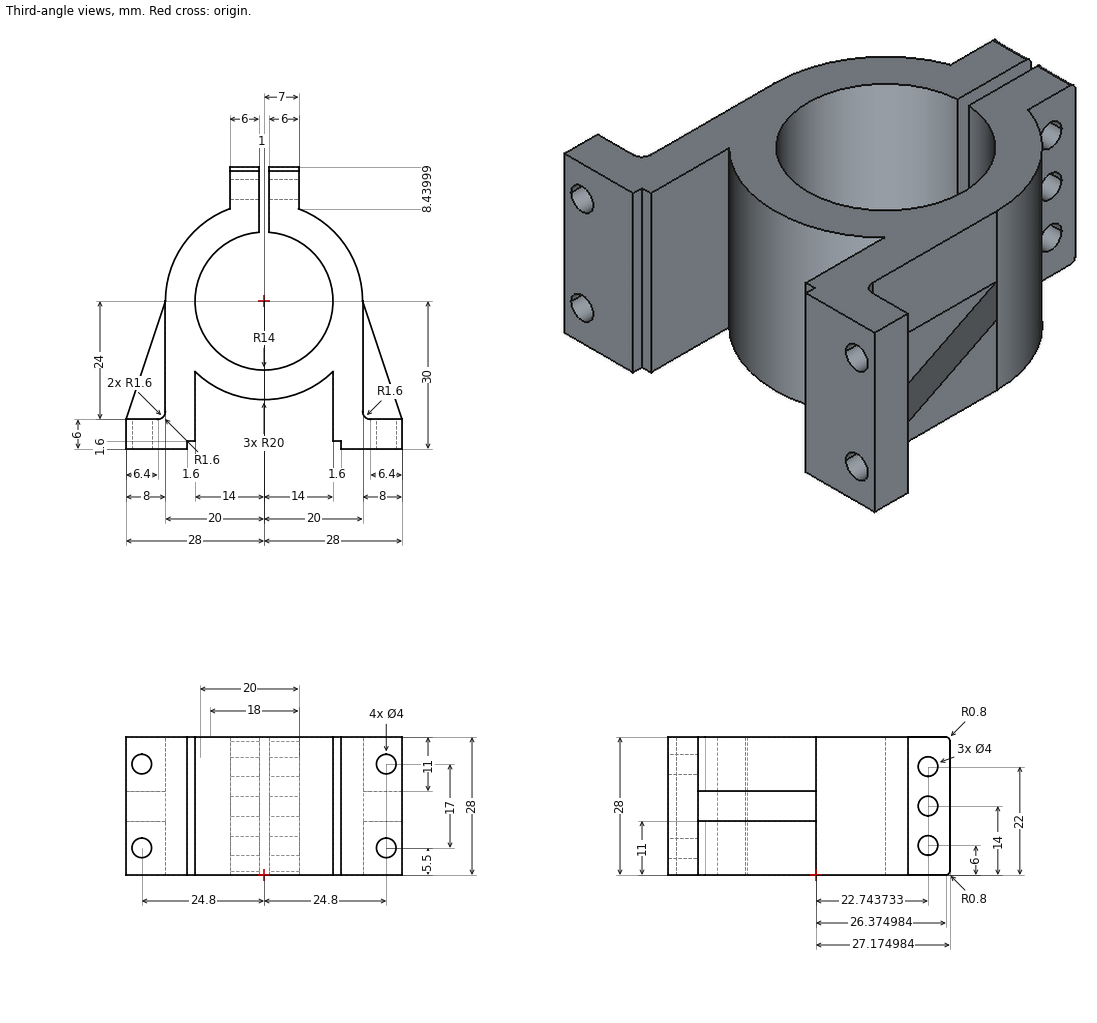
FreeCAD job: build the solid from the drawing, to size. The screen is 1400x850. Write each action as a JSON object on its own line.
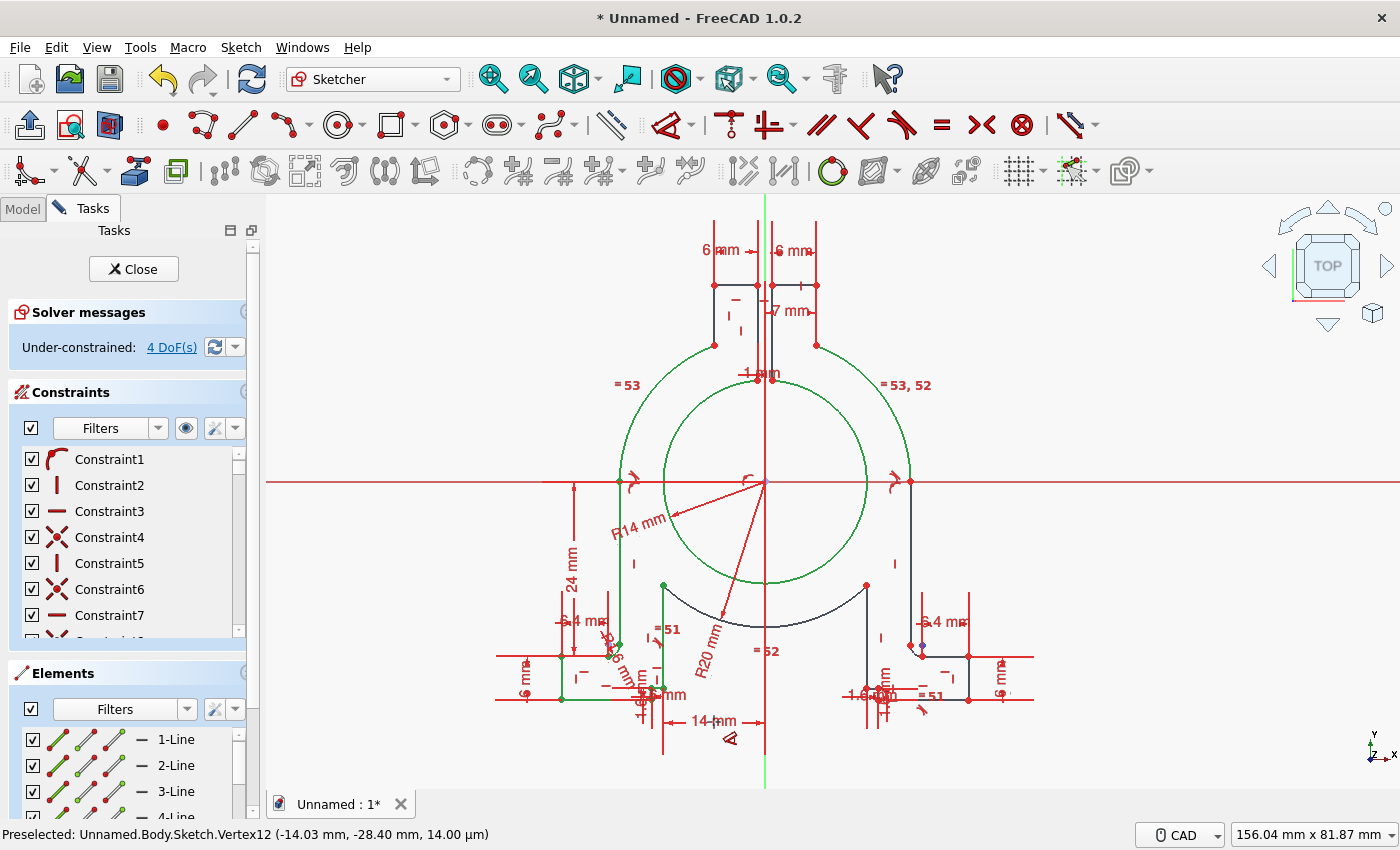
{"action": "left_click", "coordinate": [867, 586]}
{"action": "left_click", "coordinate": [852, 620]}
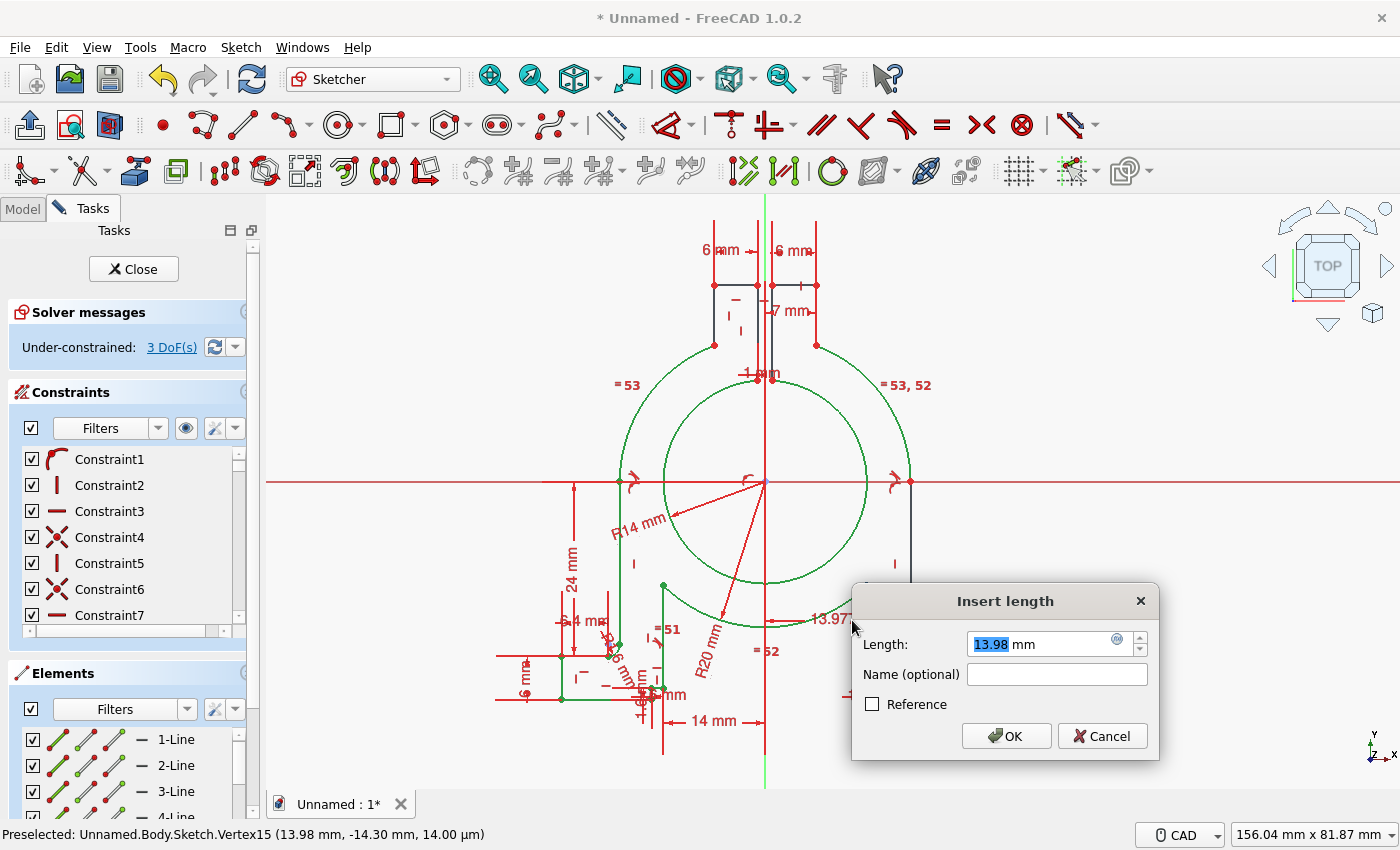
{"action": "type", "text": "14"}
{"action": "key", "text": "Return"}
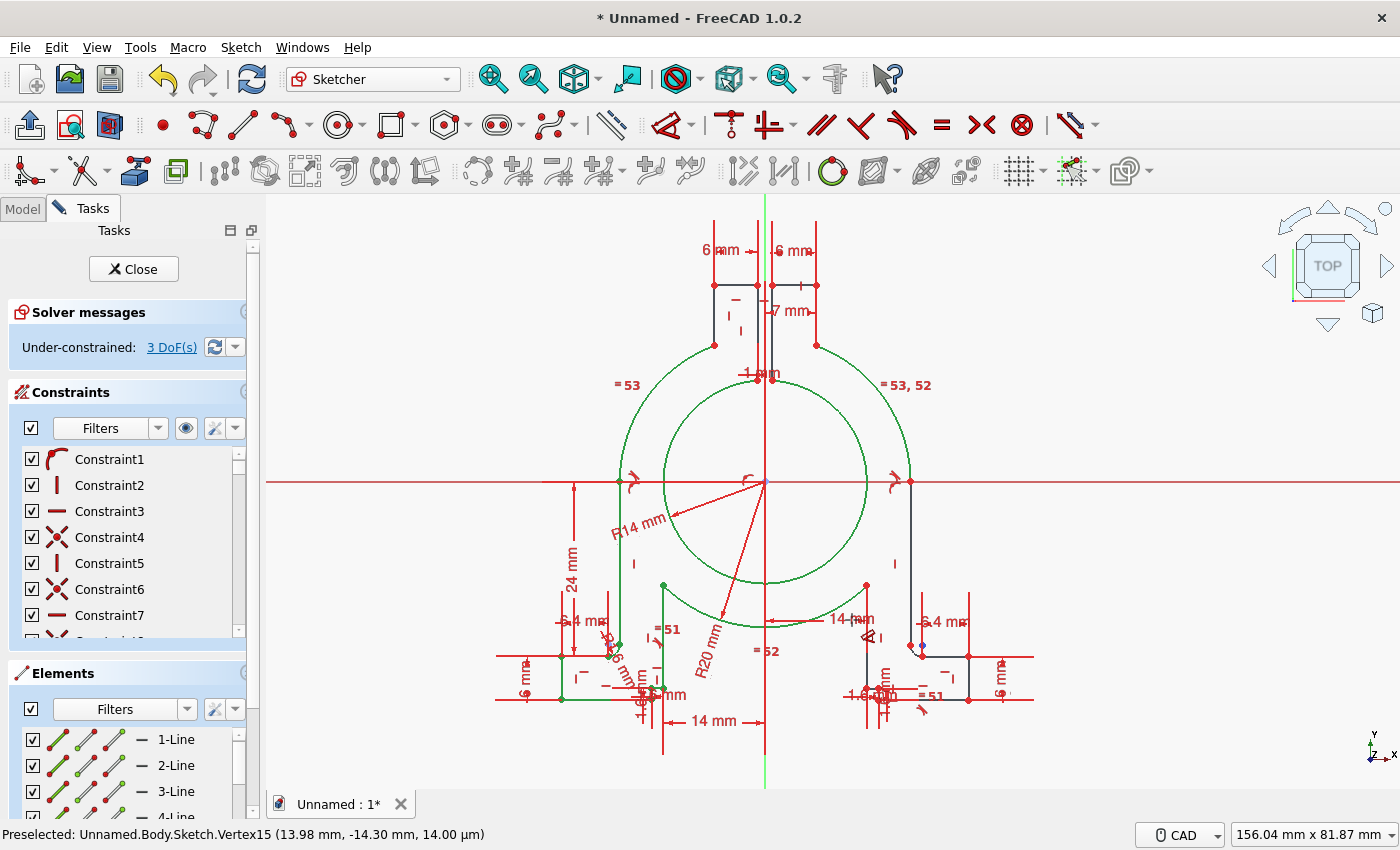
{"action": "left_click", "coordinate": [879, 700]}
{"action": "left_click", "coordinate": [731, 541]}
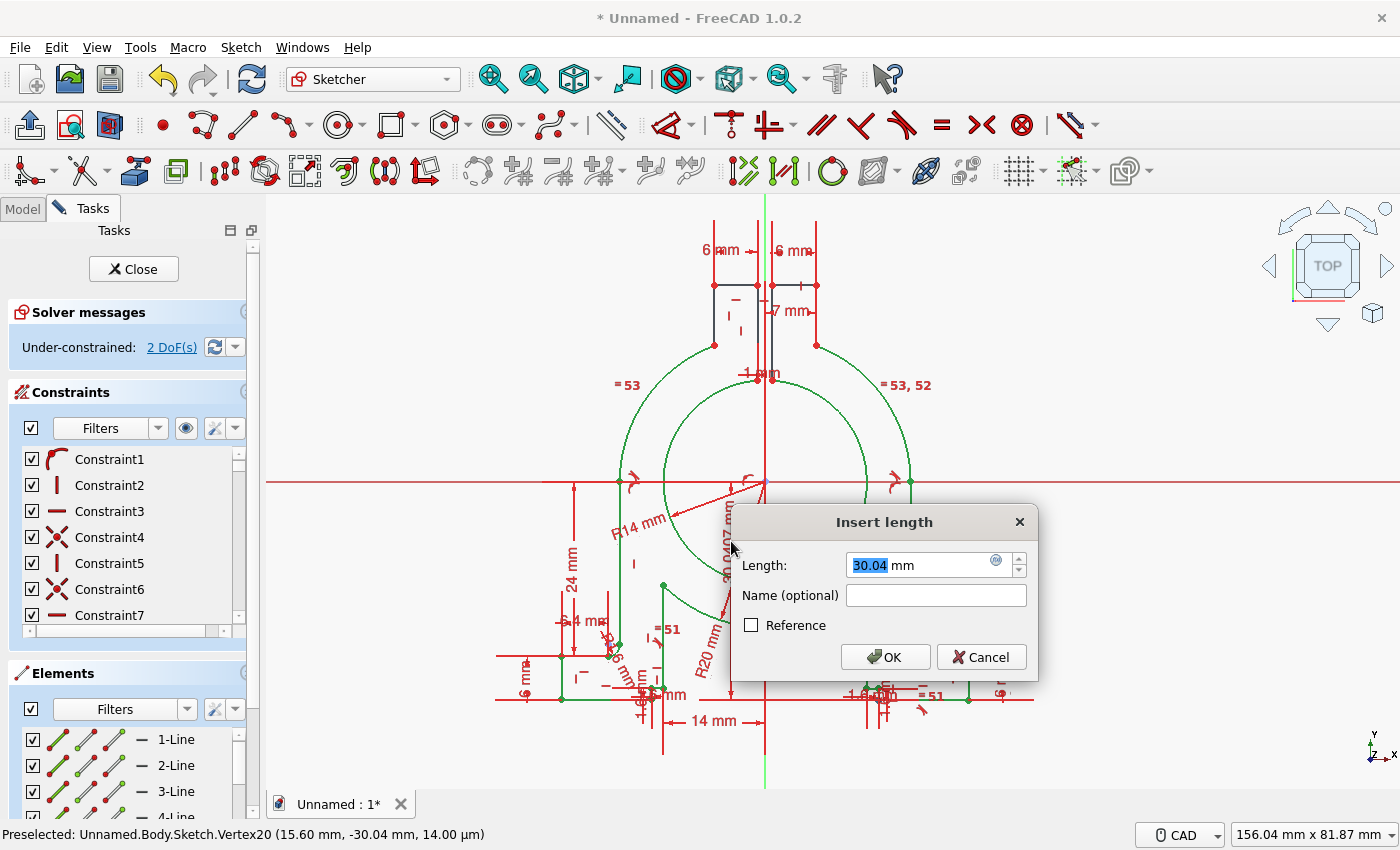
{"action": "type", "text": "30"}
{"action": "key", "text": "Return"}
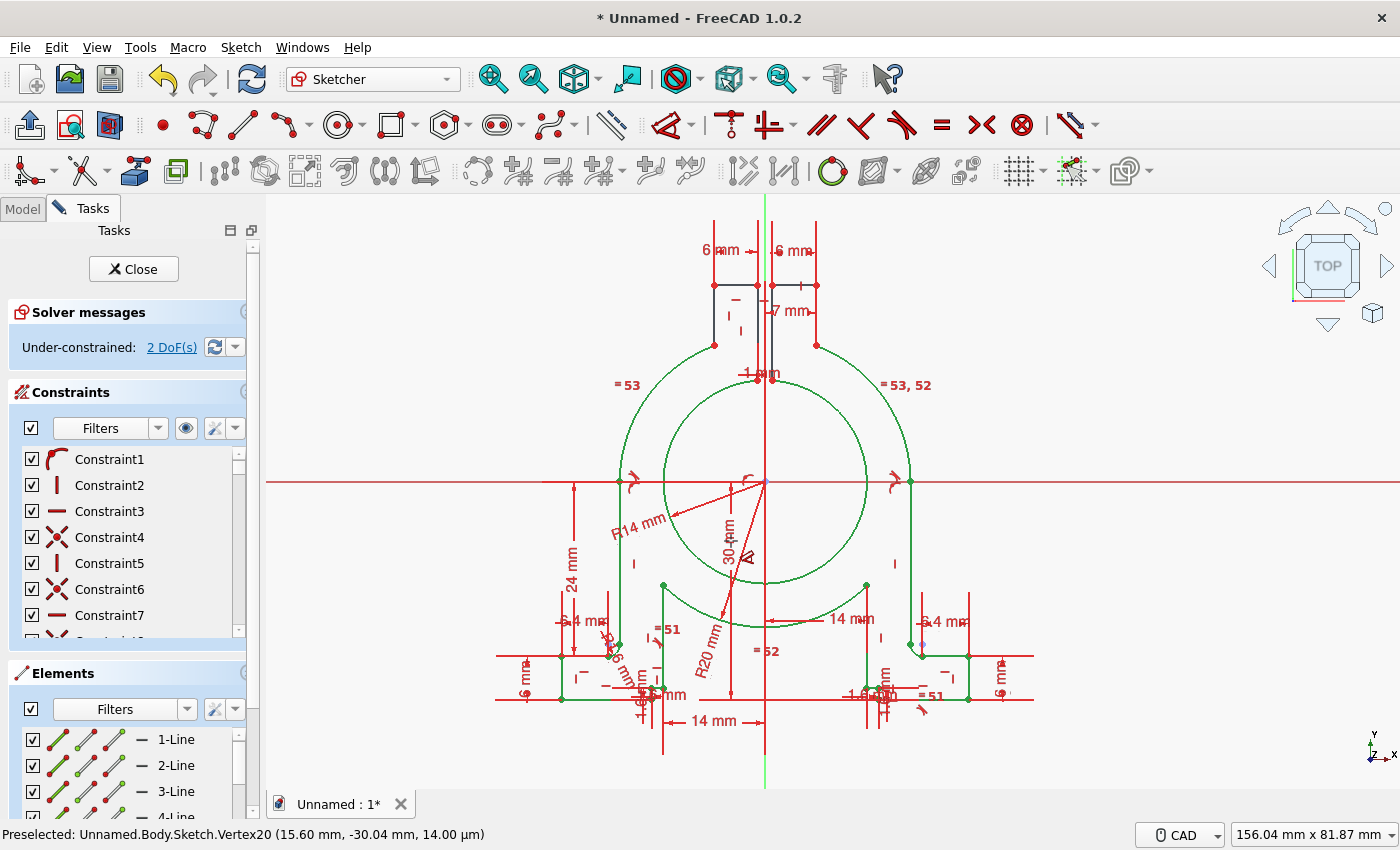
{"action": "left_click", "coordinate": [816, 328]}
{"action": "left_click", "coordinate": [850, 337]}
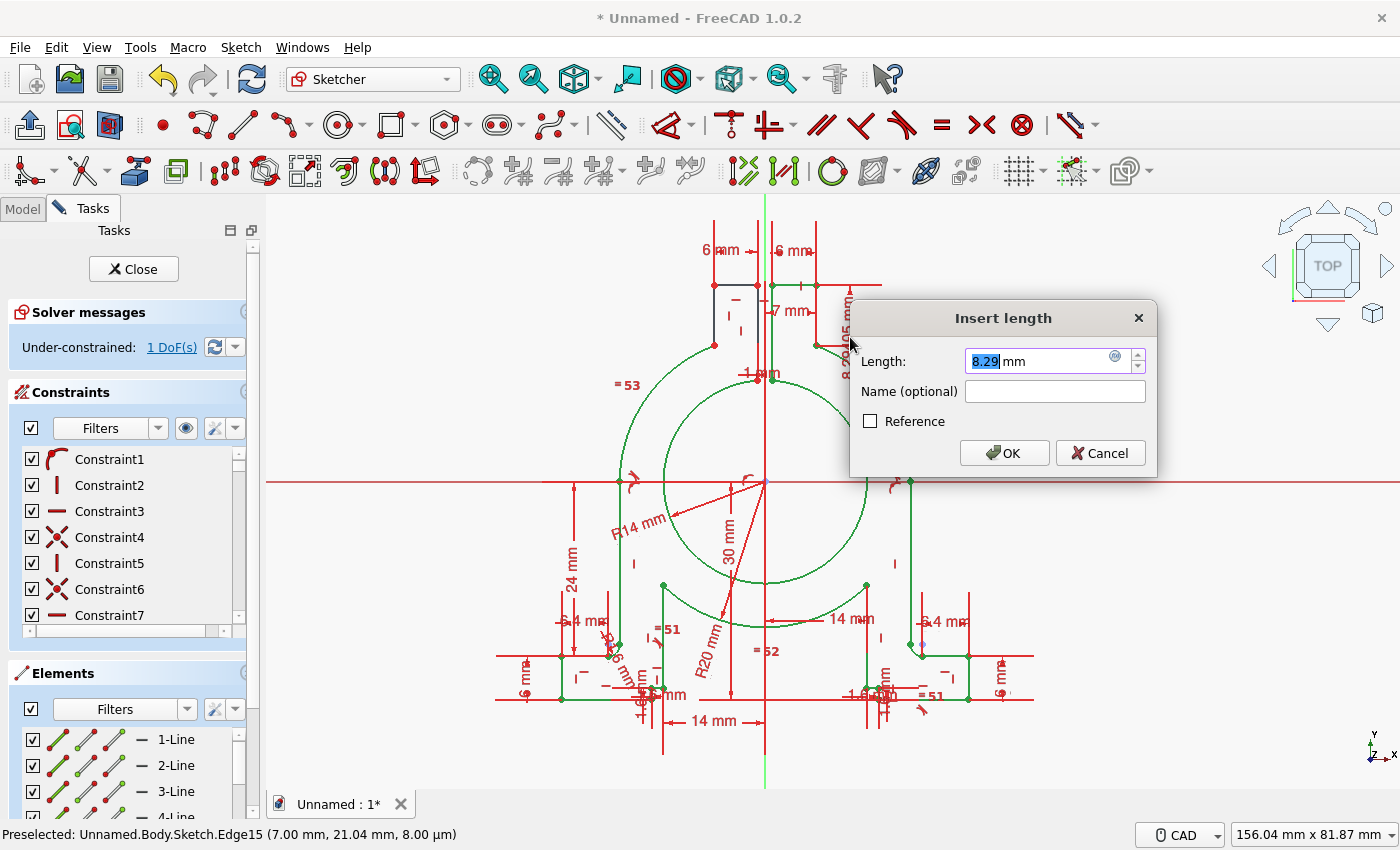
{"action": "type", "text": "8.43999"}
{"action": "key", "text": "Return"}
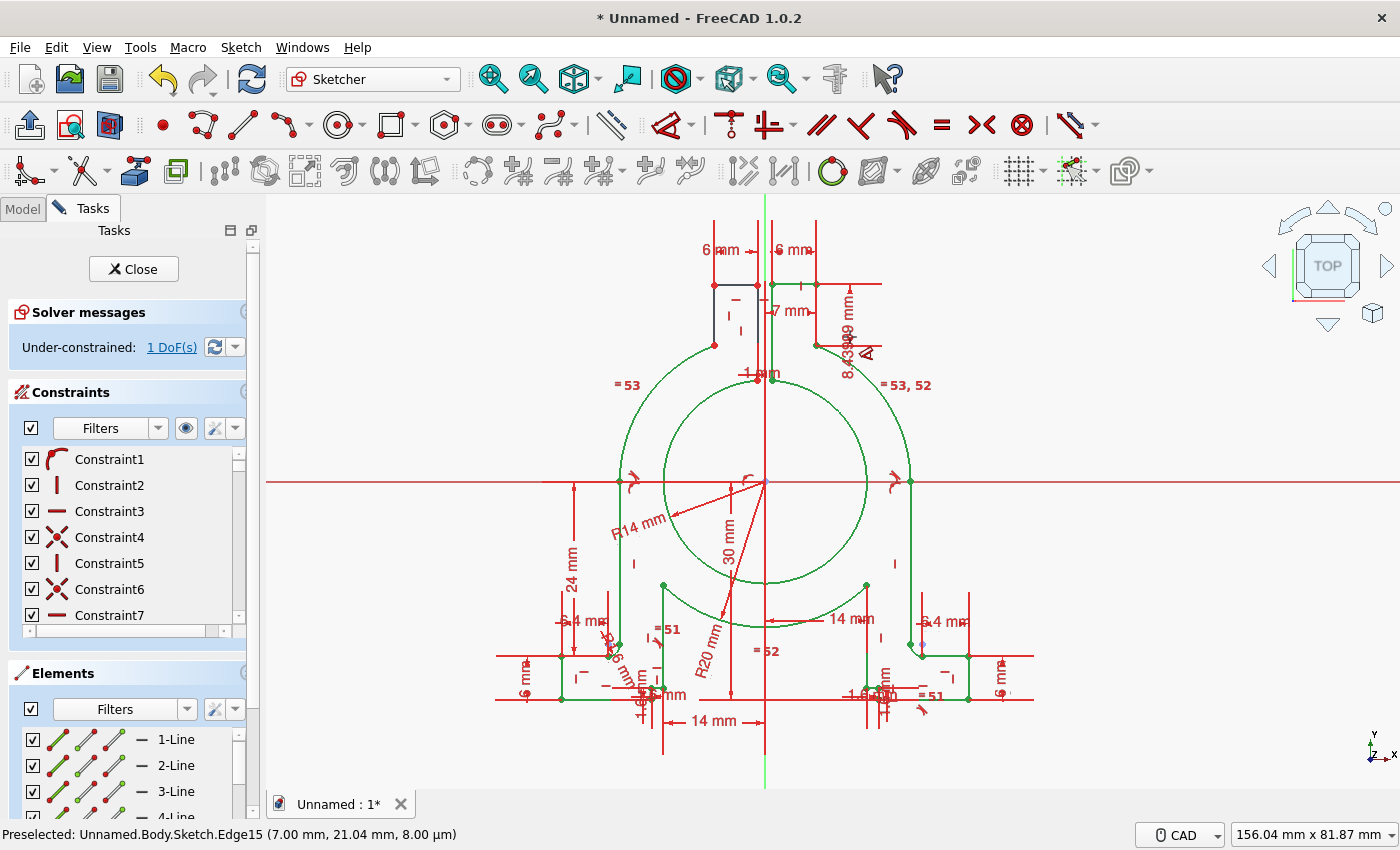
{"action": "left_click", "coordinate": [714, 303]}
{"action": "left_click", "coordinate": [680, 315]}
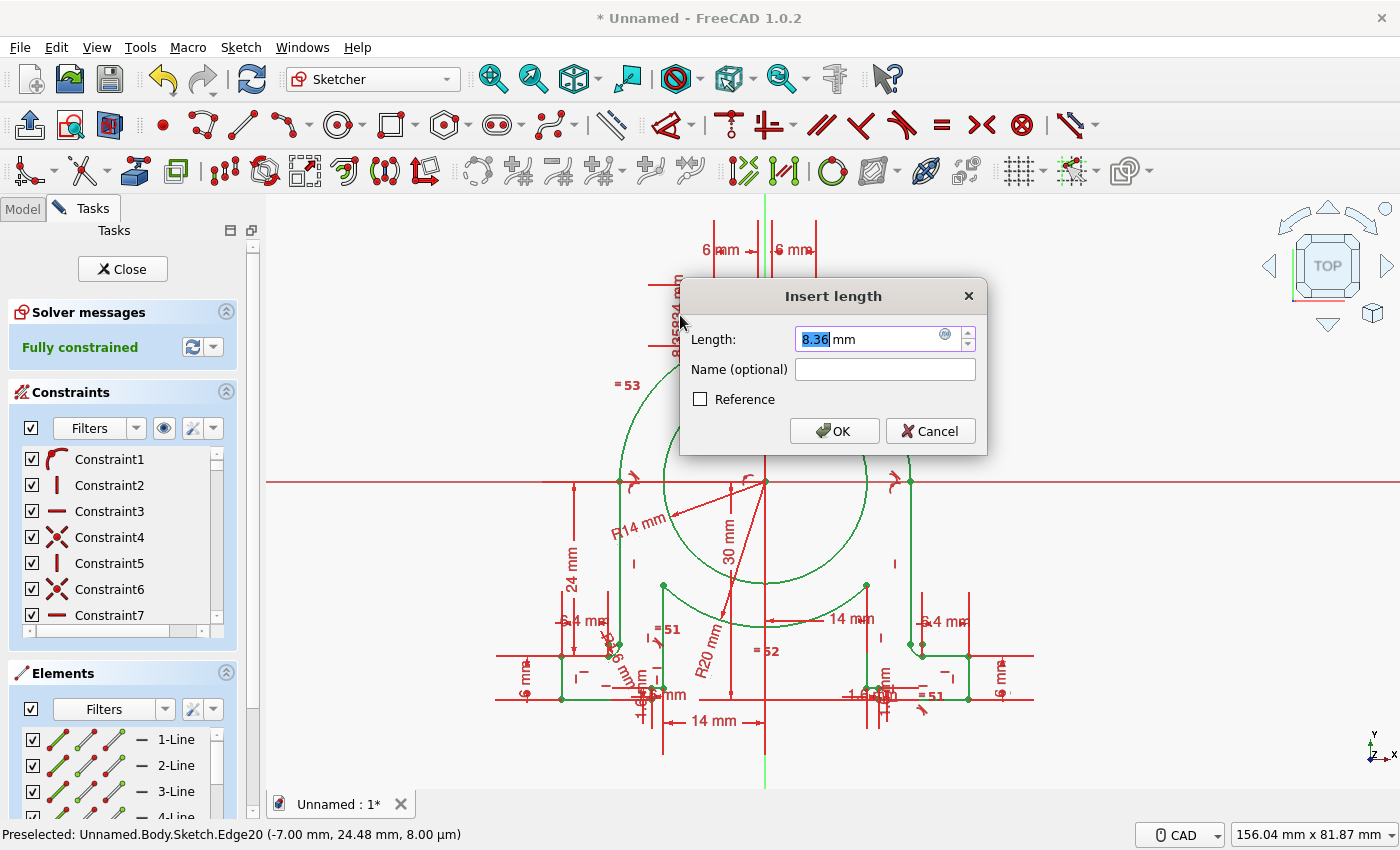
{"action": "type", "text": "8.43999"}
{"action": "key", "text": "Return"}
{"action": "key", "text": "Escape"}